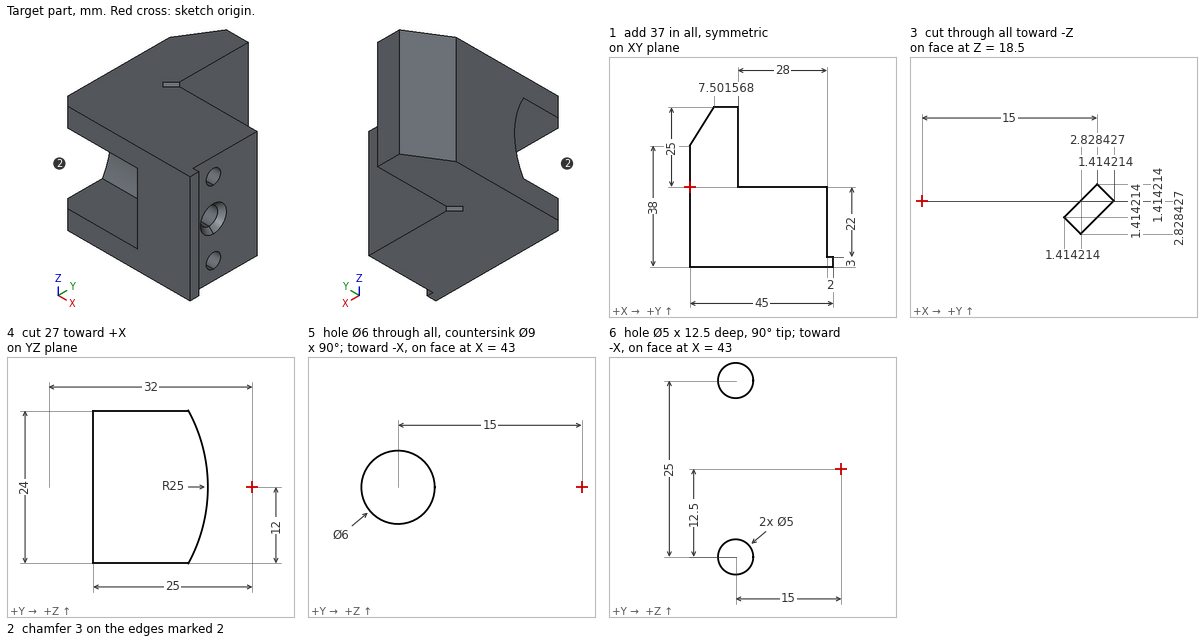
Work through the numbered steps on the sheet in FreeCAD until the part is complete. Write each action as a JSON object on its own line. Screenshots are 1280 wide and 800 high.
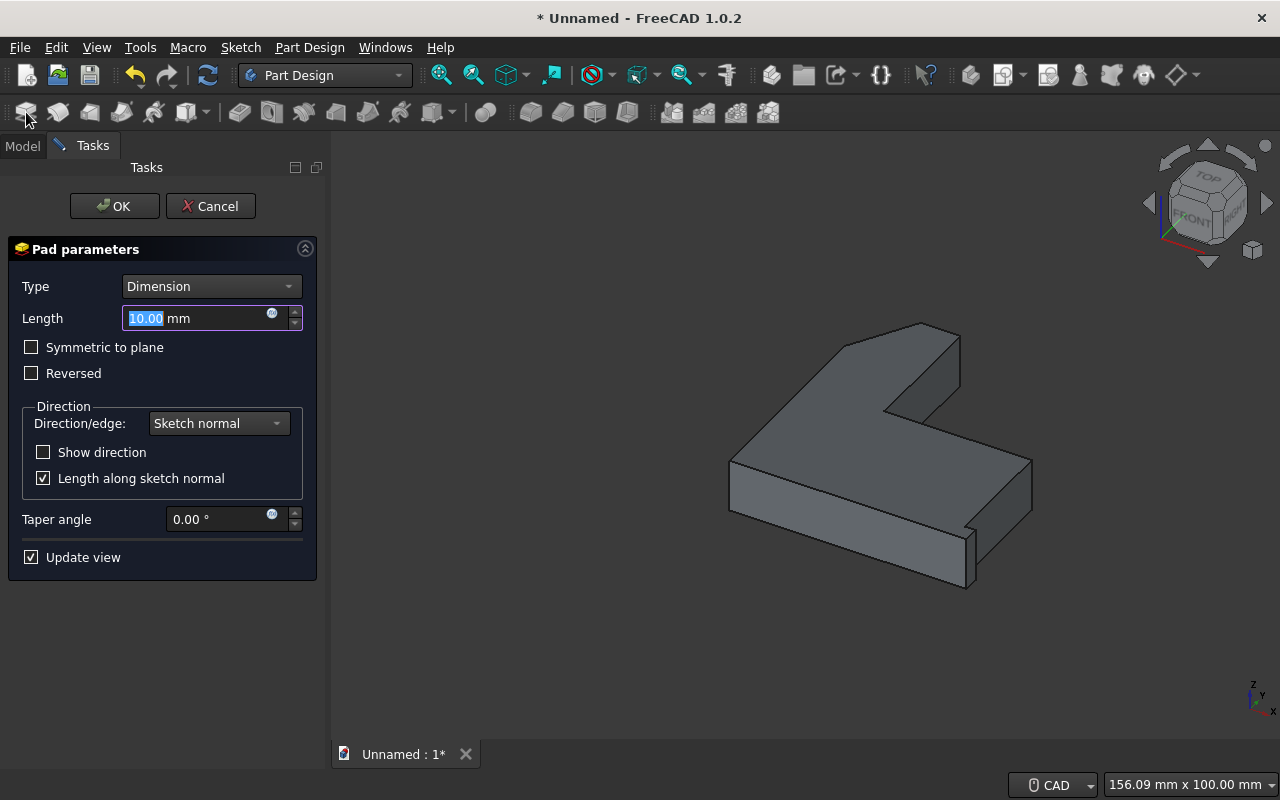
{"action": "type", "text": "37"}
{"action": "key", "text": "Tab"}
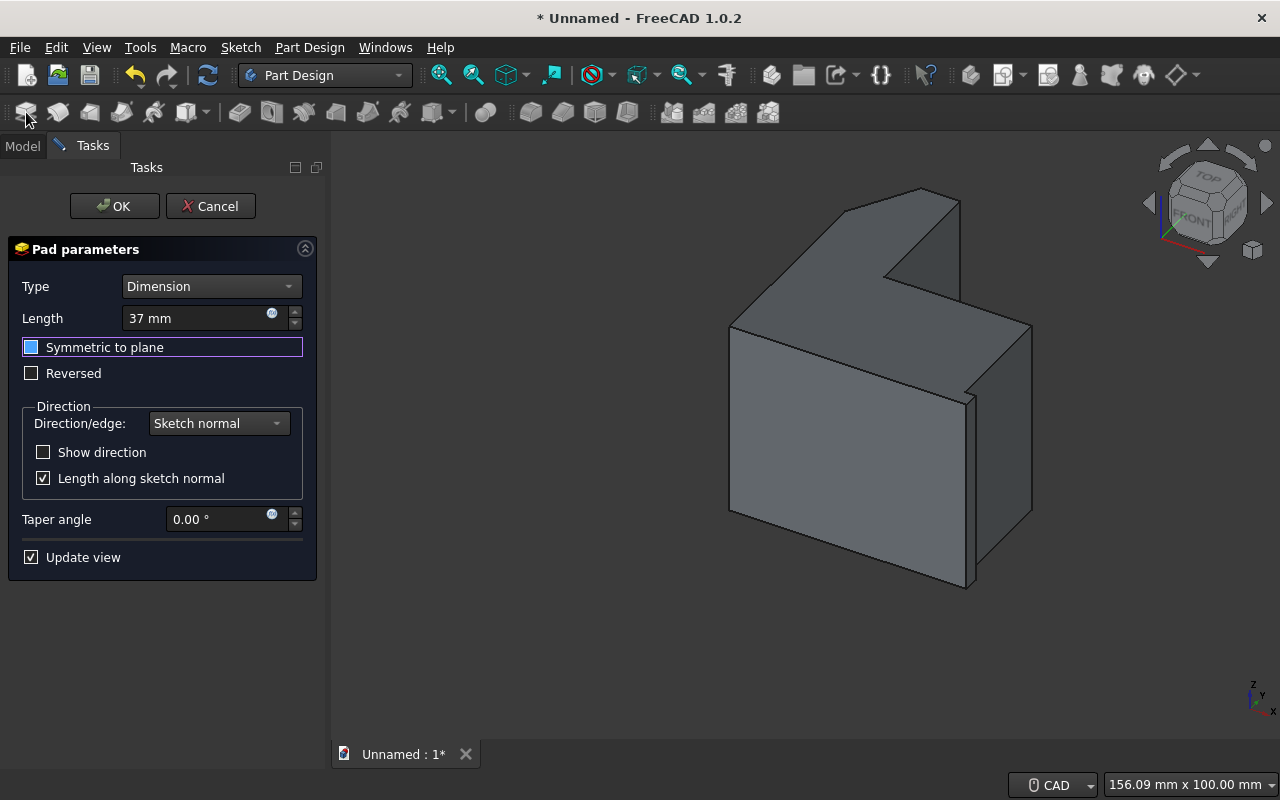
{"action": "left_click", "coordinate": [30, 347]}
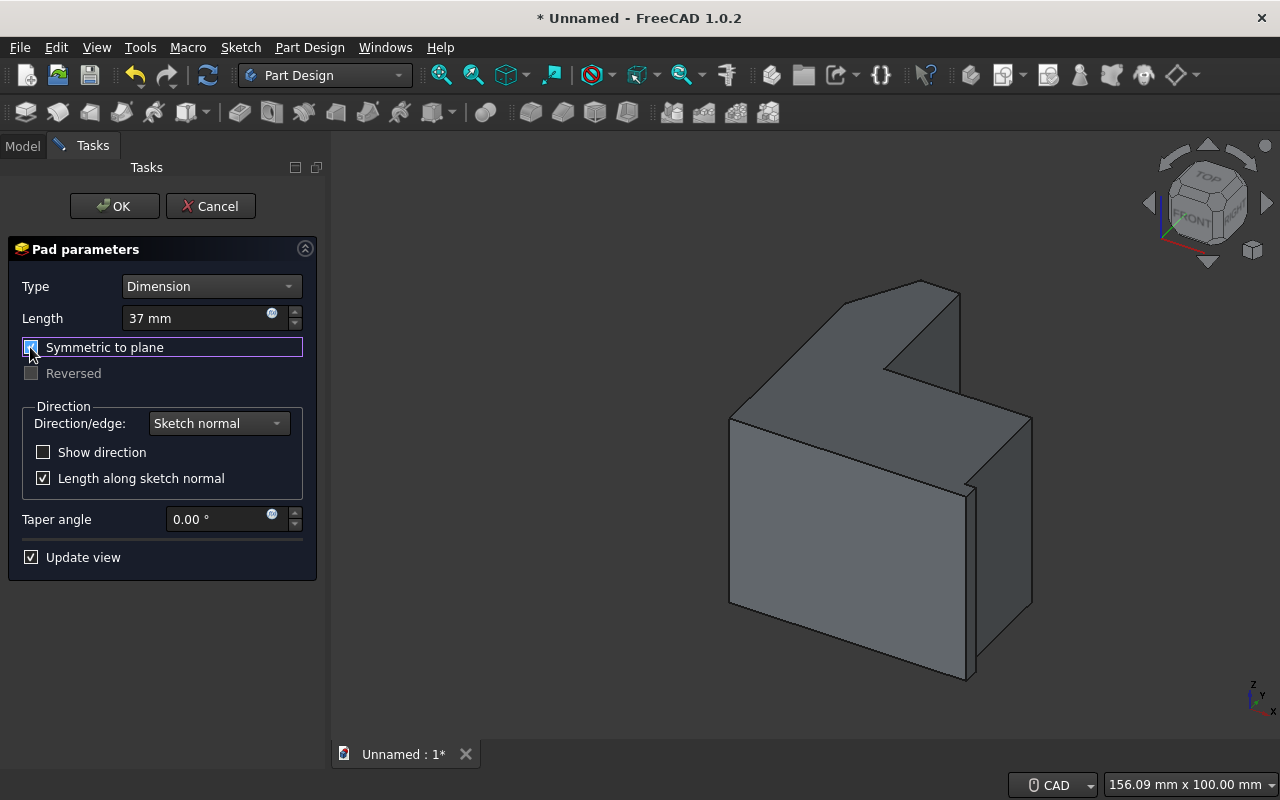
{"action": "left_click", "coordinate": [115, 206]}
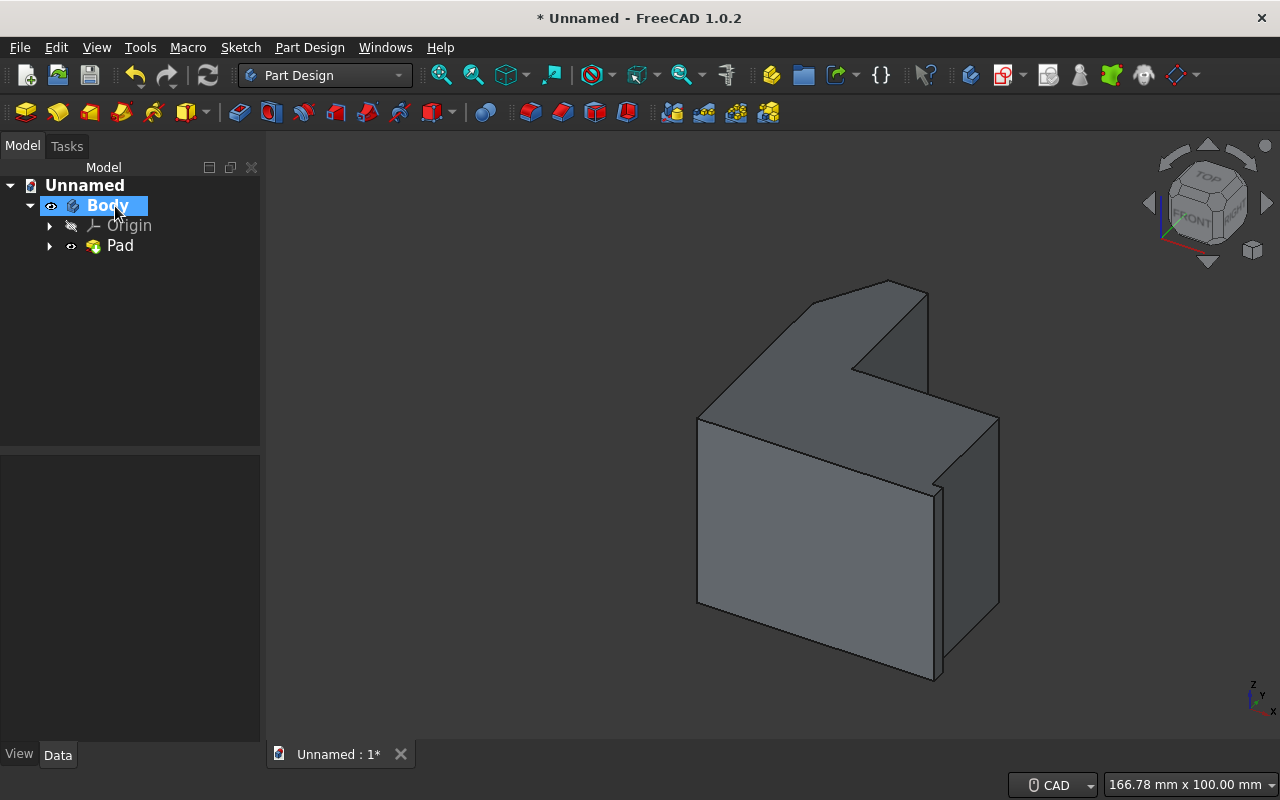
{"action": "key", "text": "0"}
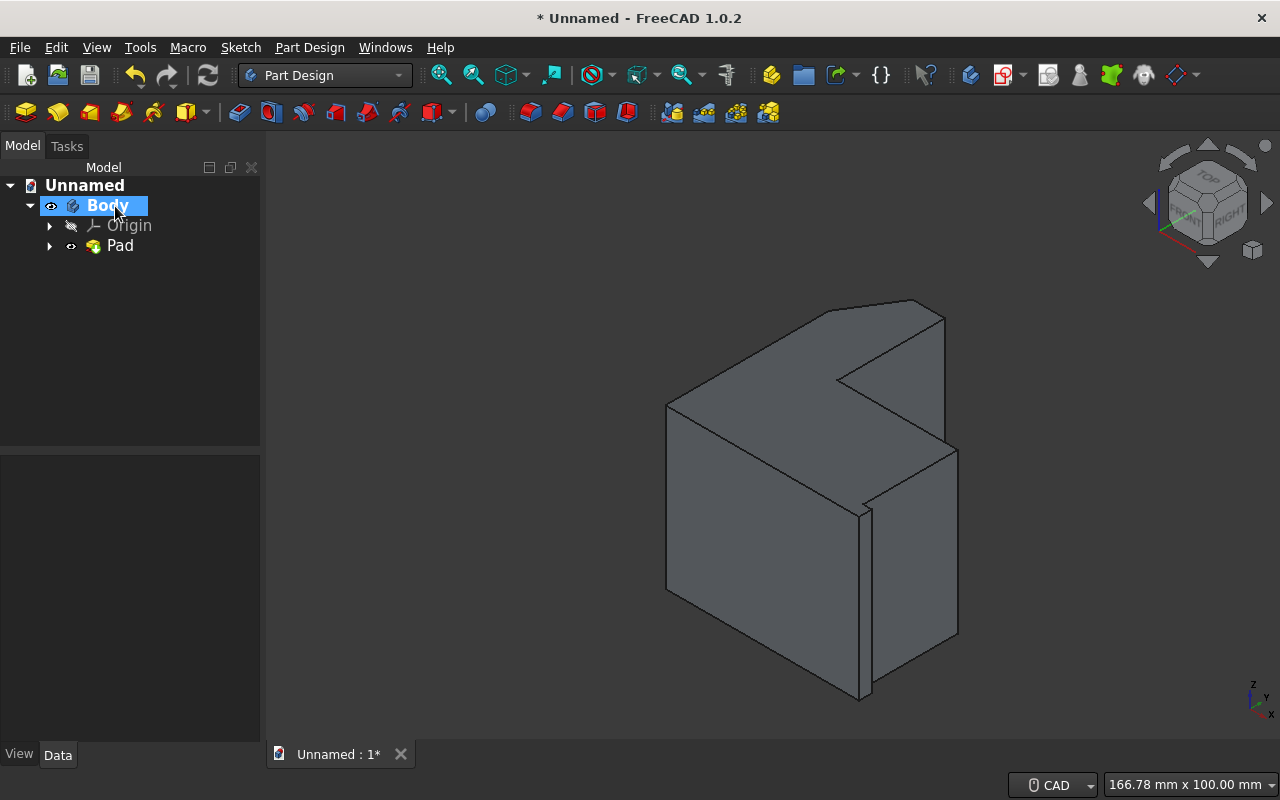
{"action": "key", "text": "2"}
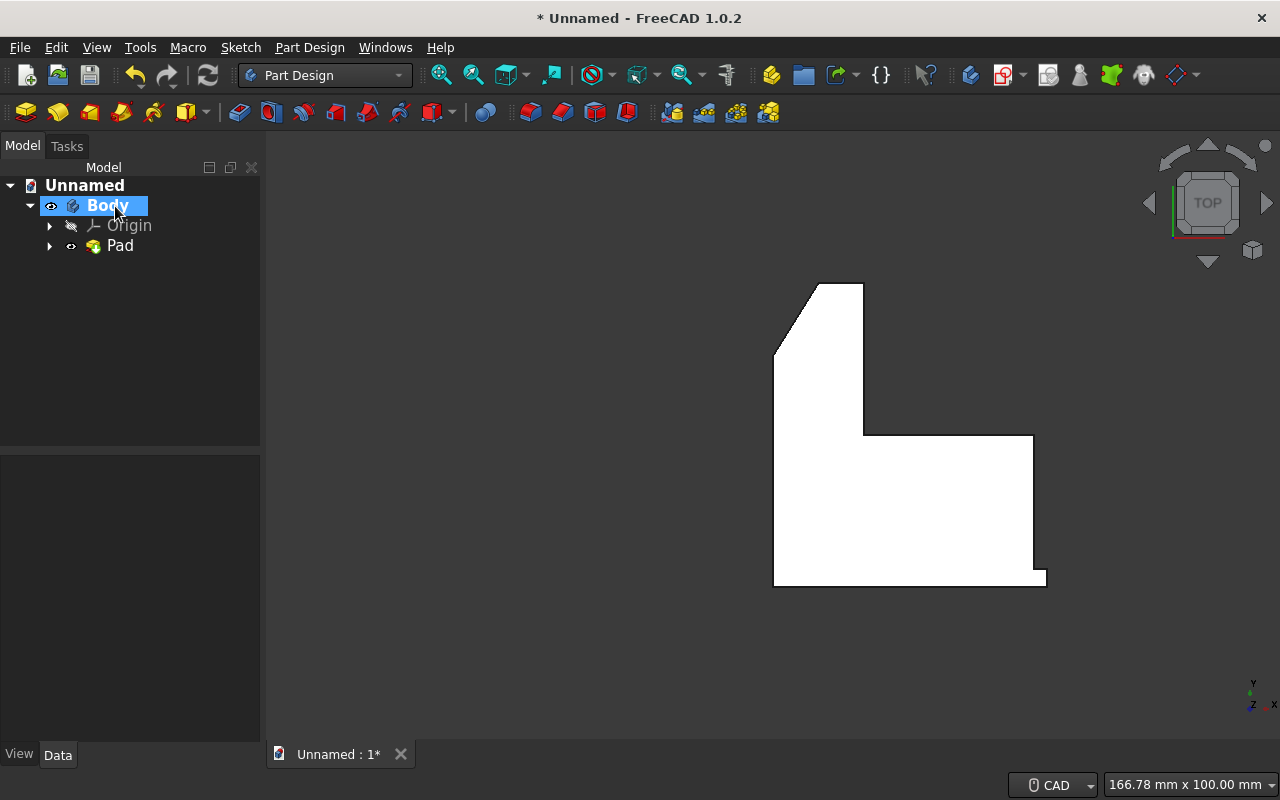
{"action": "key", "text": "1"}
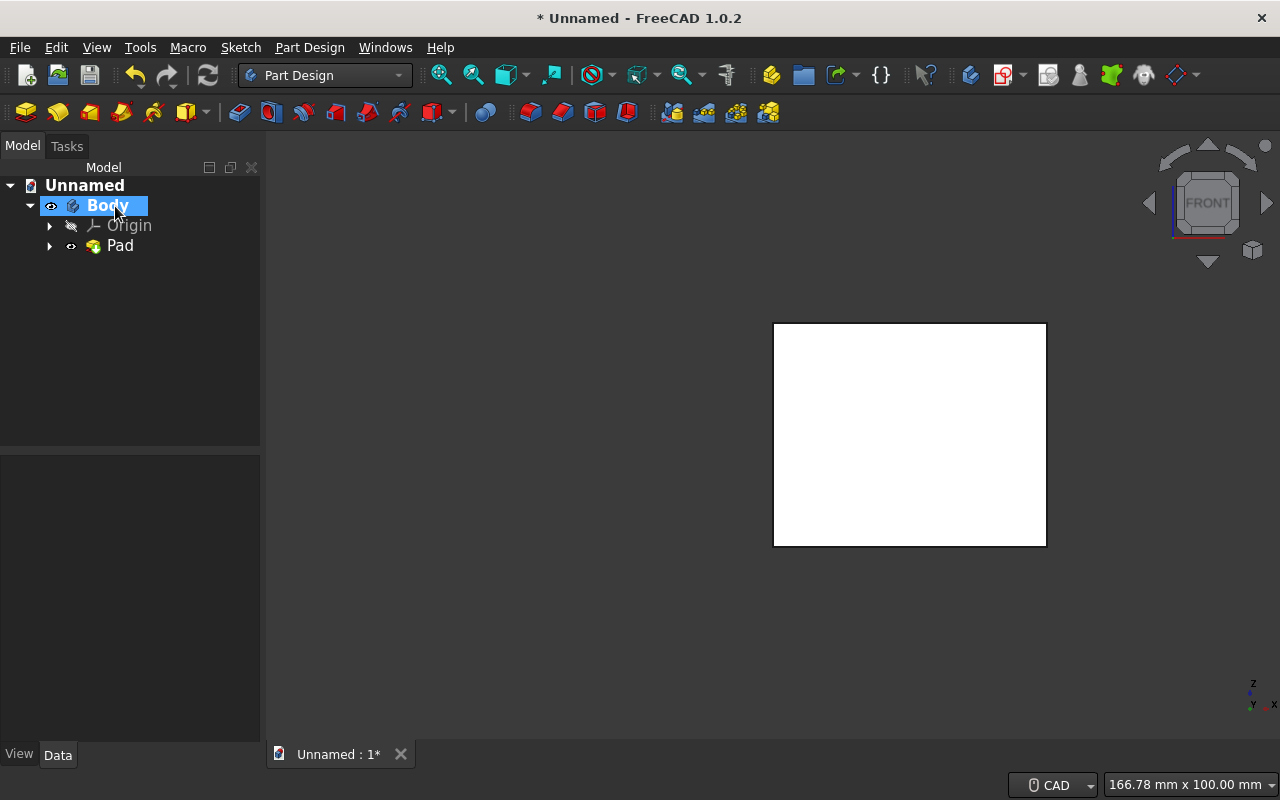
{"action": "left_click", "coordinate": [442, 76]}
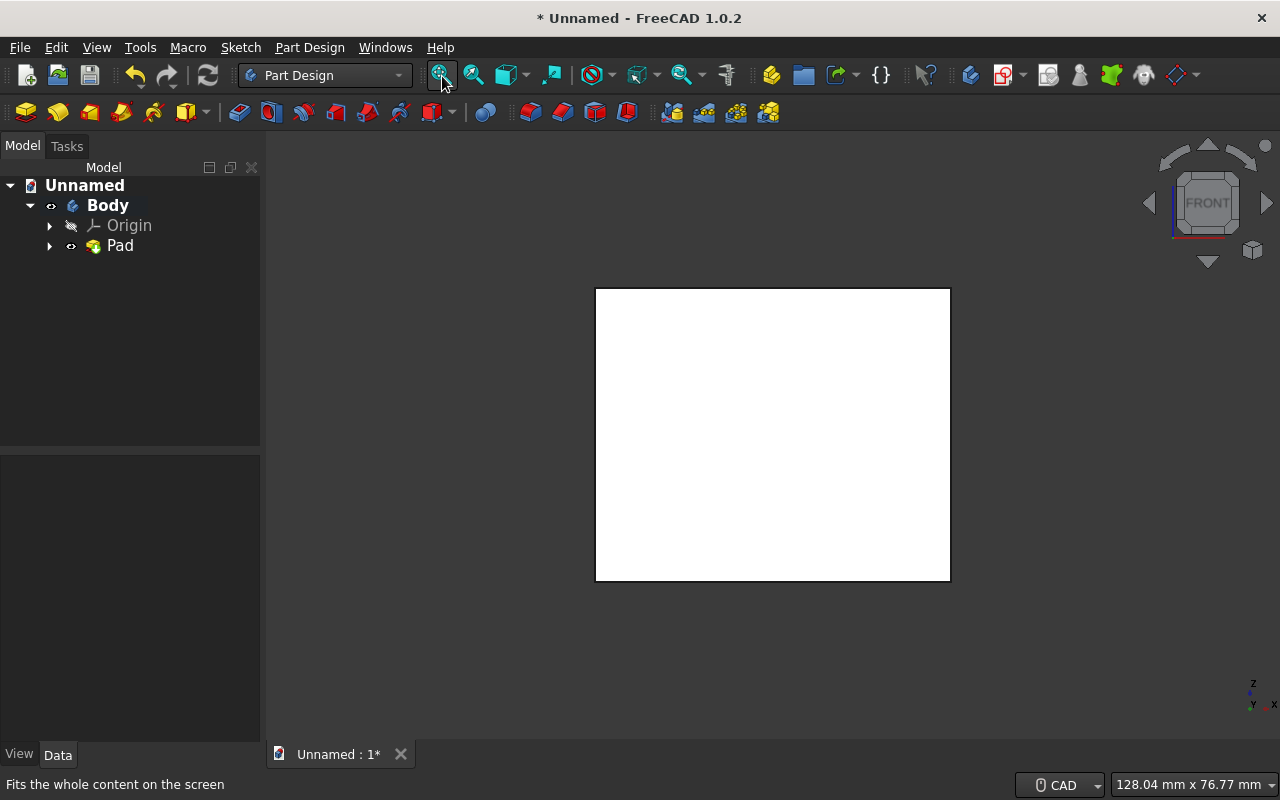
{"action": "left_click", "coordinate": [595, 434]}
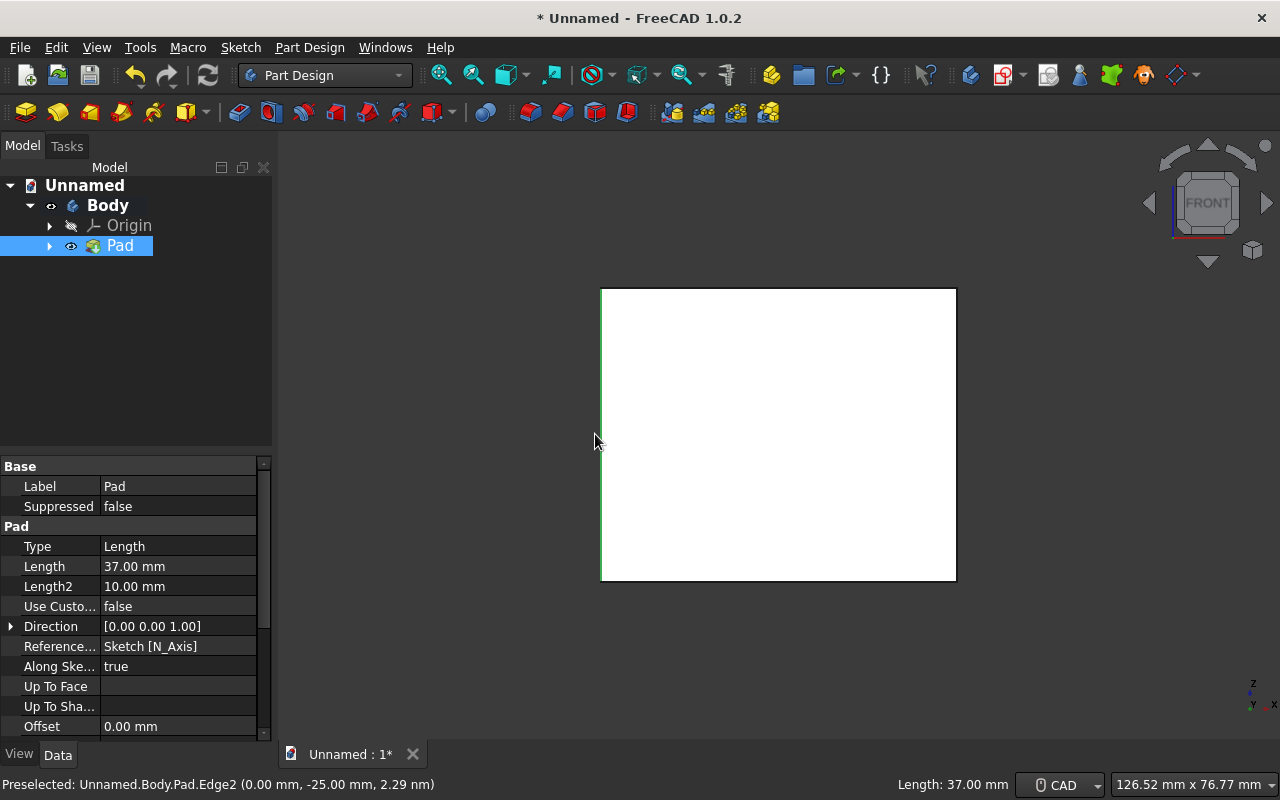
{"action": "left_click", "coordinate": [564, 112]}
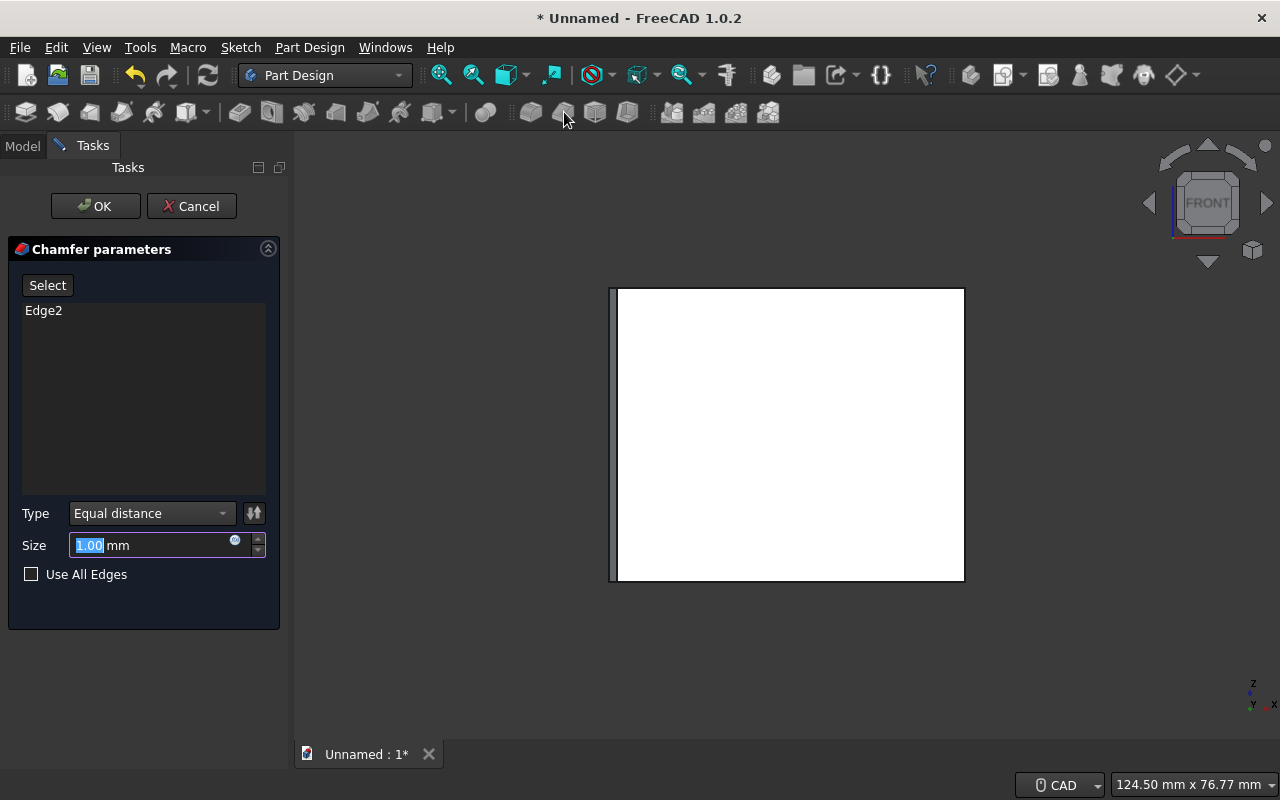
{"action": "type", "text": "3"}
{"action": "key", "text": "Tab"}